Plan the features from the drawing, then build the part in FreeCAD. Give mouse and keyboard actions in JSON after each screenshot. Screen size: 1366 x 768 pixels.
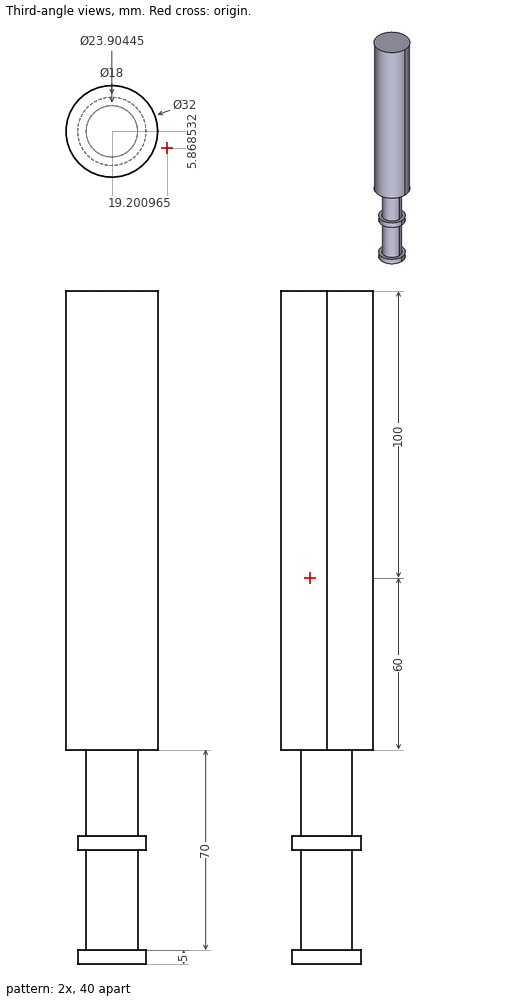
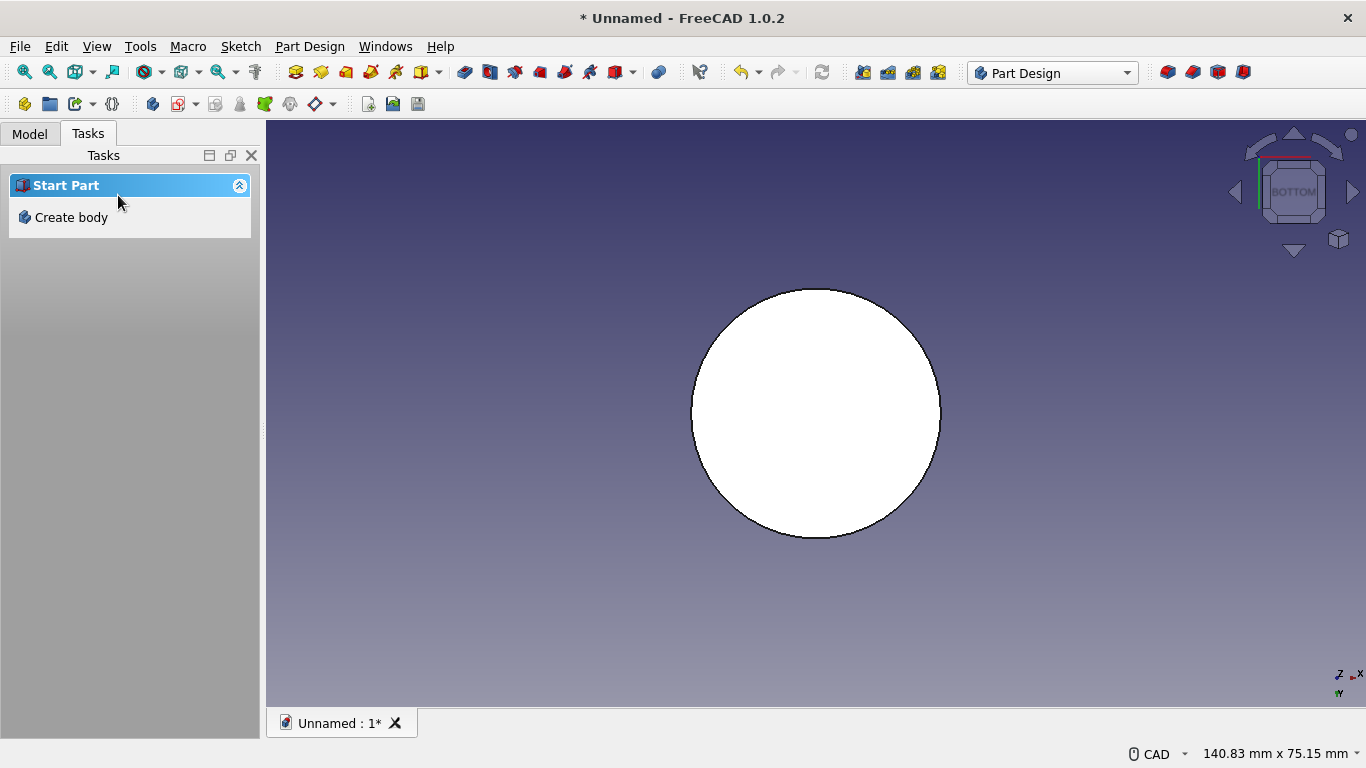
{"action": "left_click", "coordinate": [25, 72]}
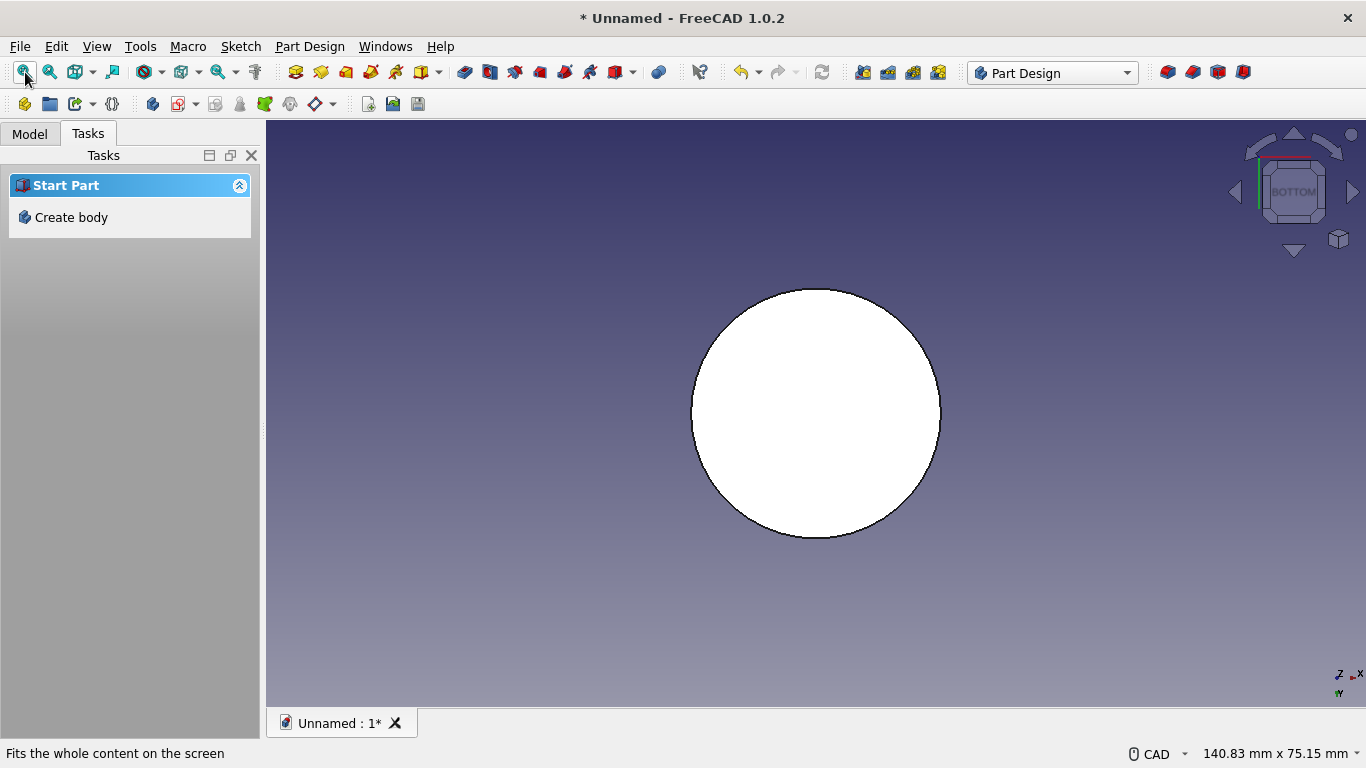
{"action": "left_click", "coordinate": [816, 412]}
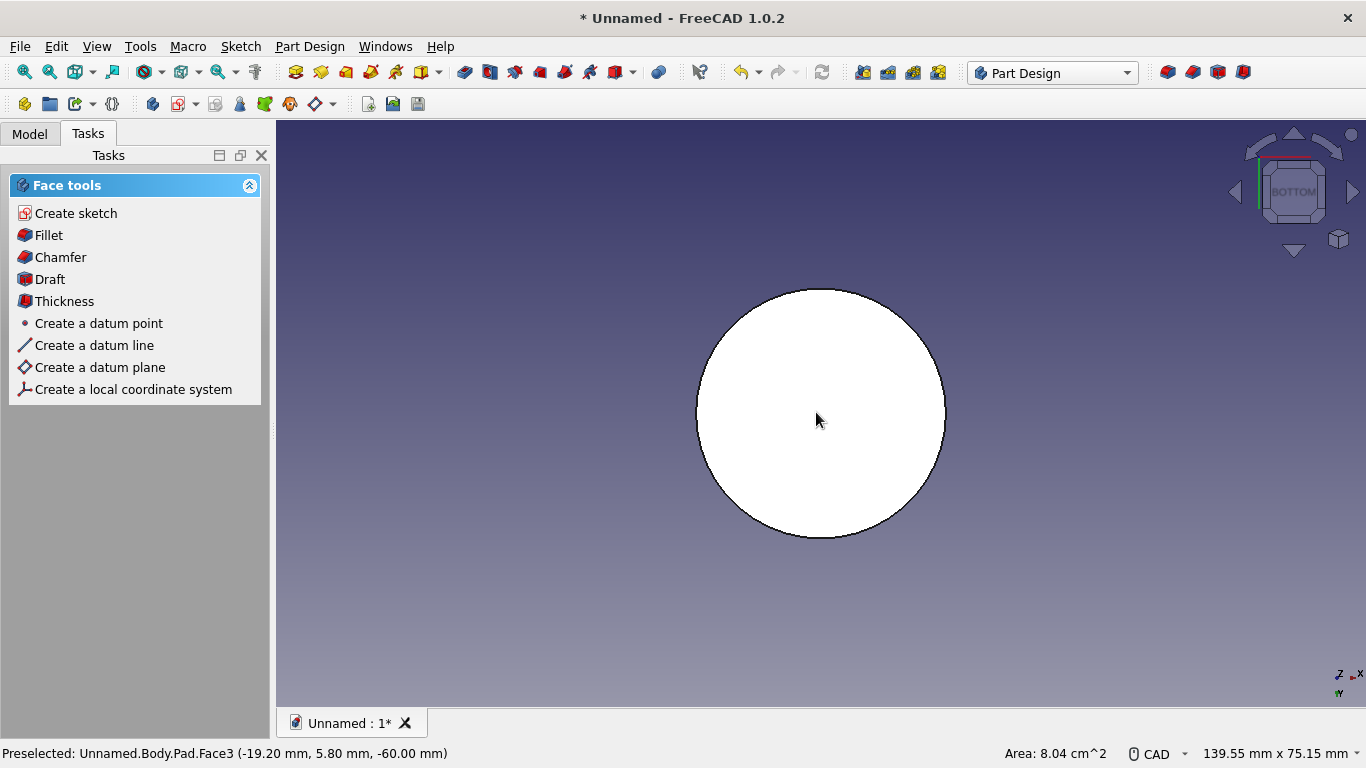
{"action": "left_click", "coordinate": [178, 104]}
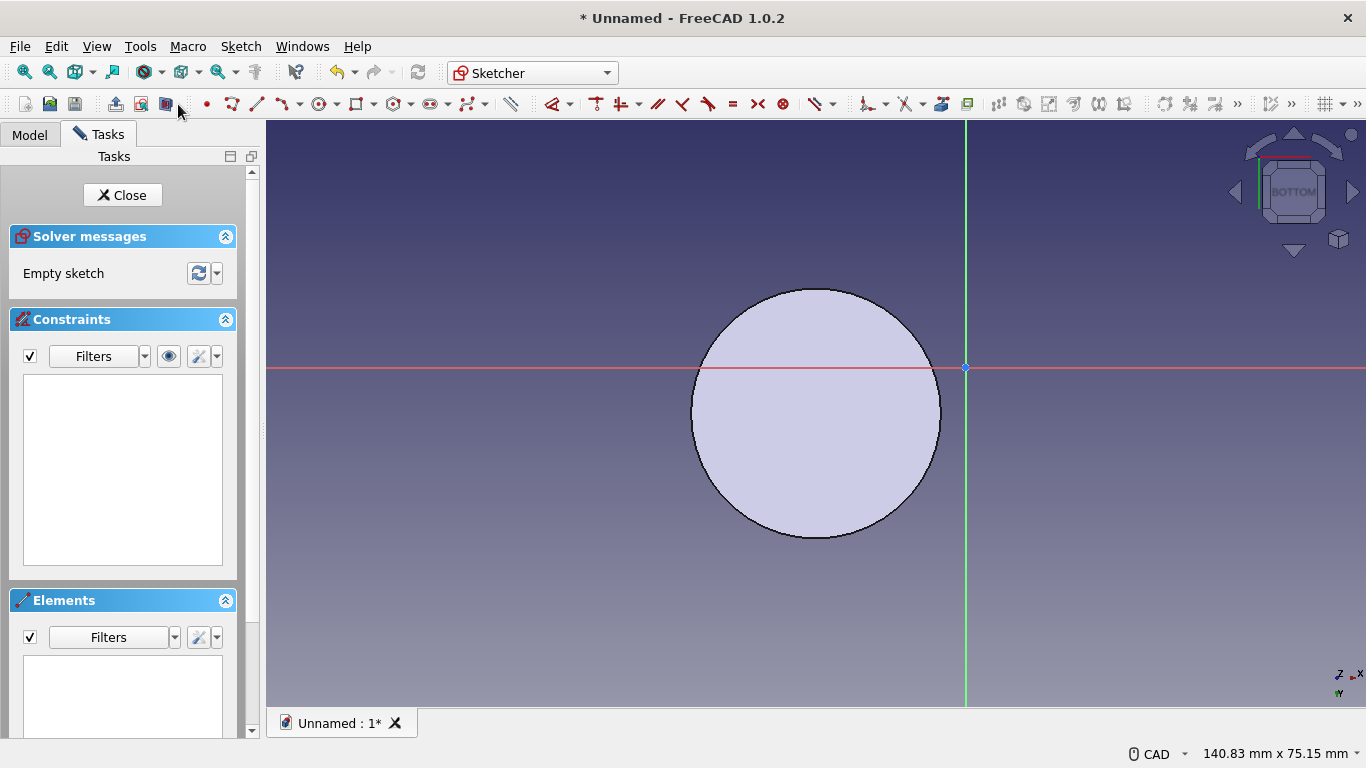
{"action": "scroll", "coordinate": [919, 413], "scroll_direction": "up", "scroll_amount": 5}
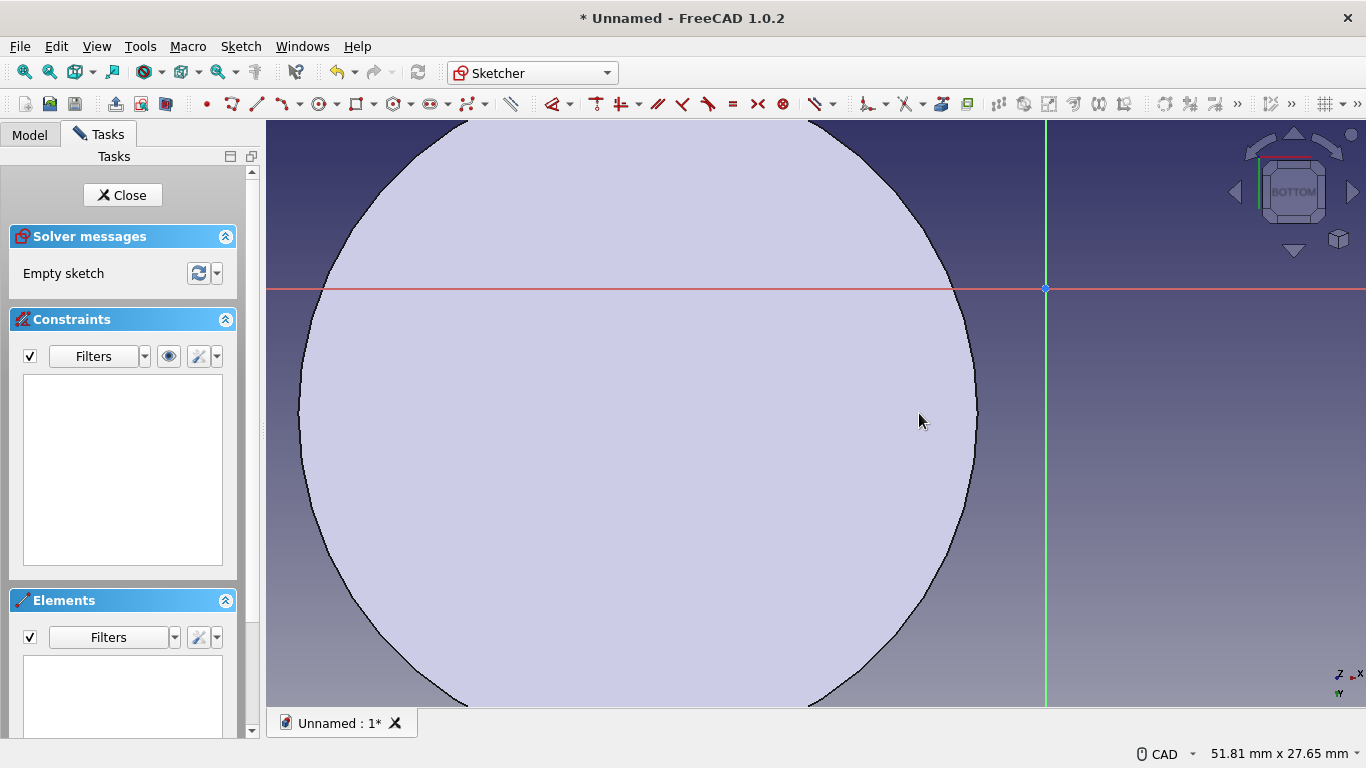
{"action": "key", "text": "g c"}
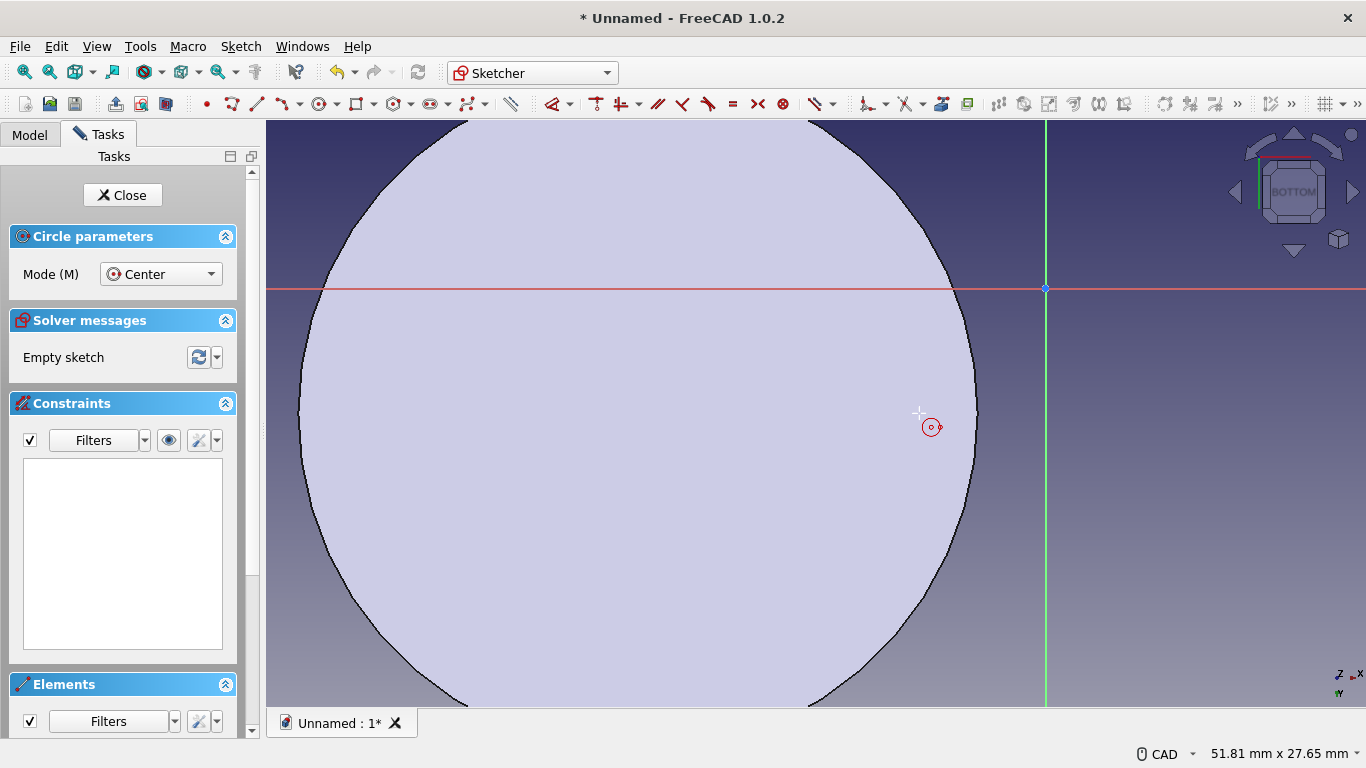
{"action": "left_click", "coordinate": [638, 413]}
{"action": "mouse_move", "coordinate": [773, 549]}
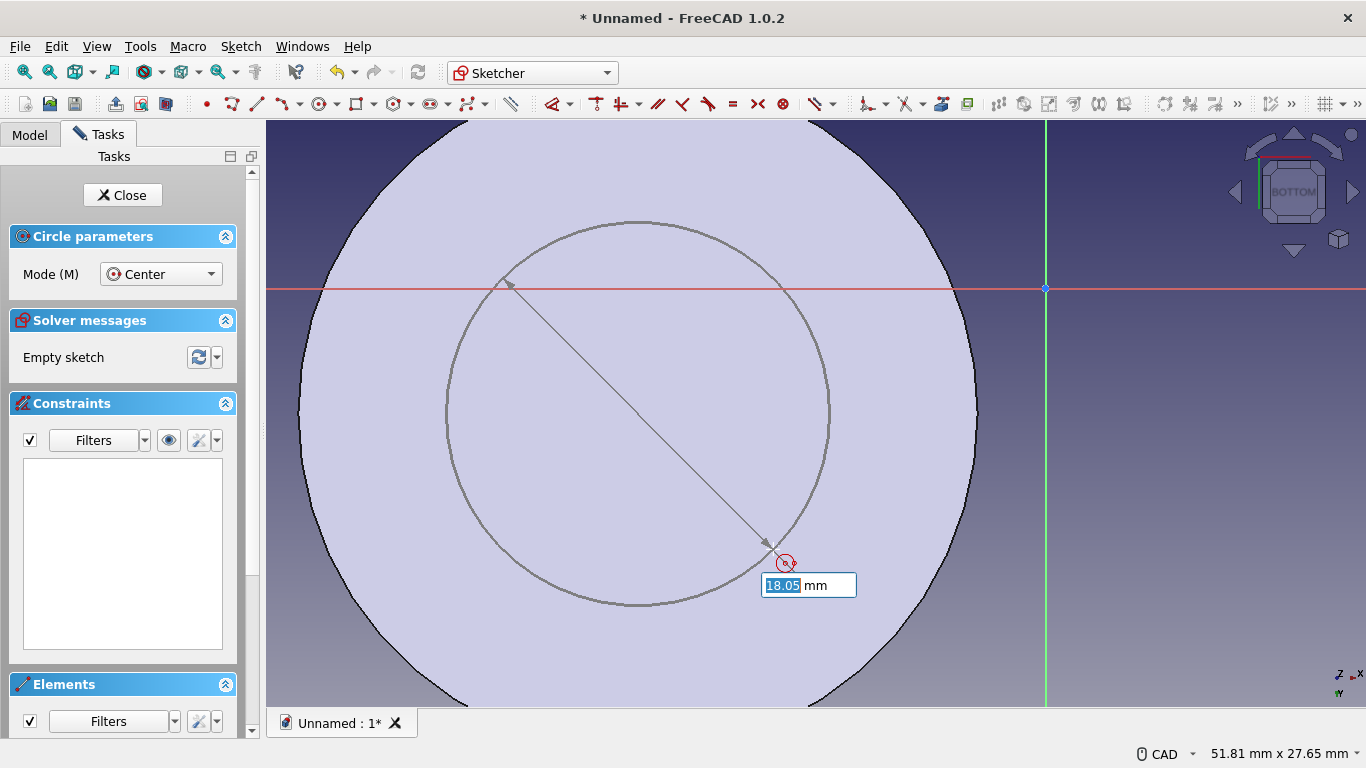
{"action": "type", "text": "18"}
{"action": "key", "text": "Return"}
{"action": "key", "text": "Escape"}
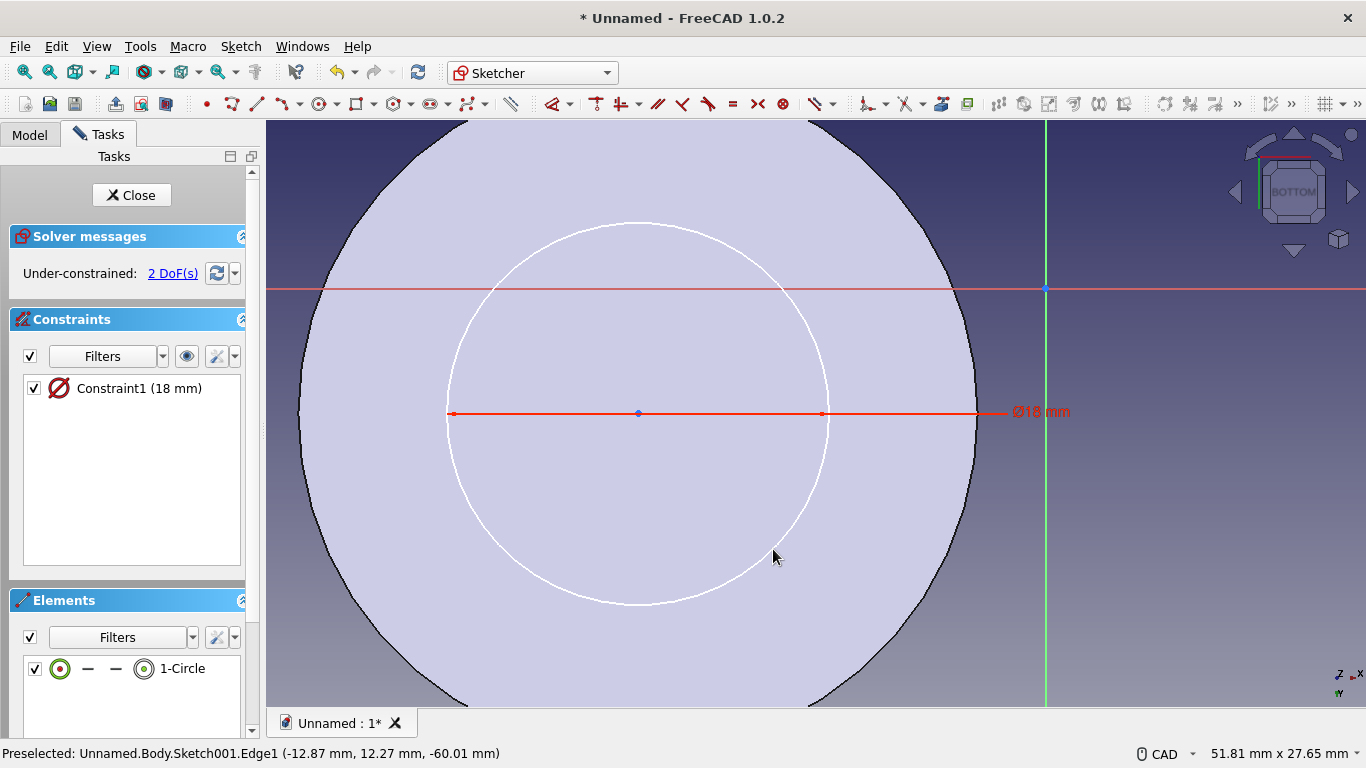
{"action": "key", "text": "d"}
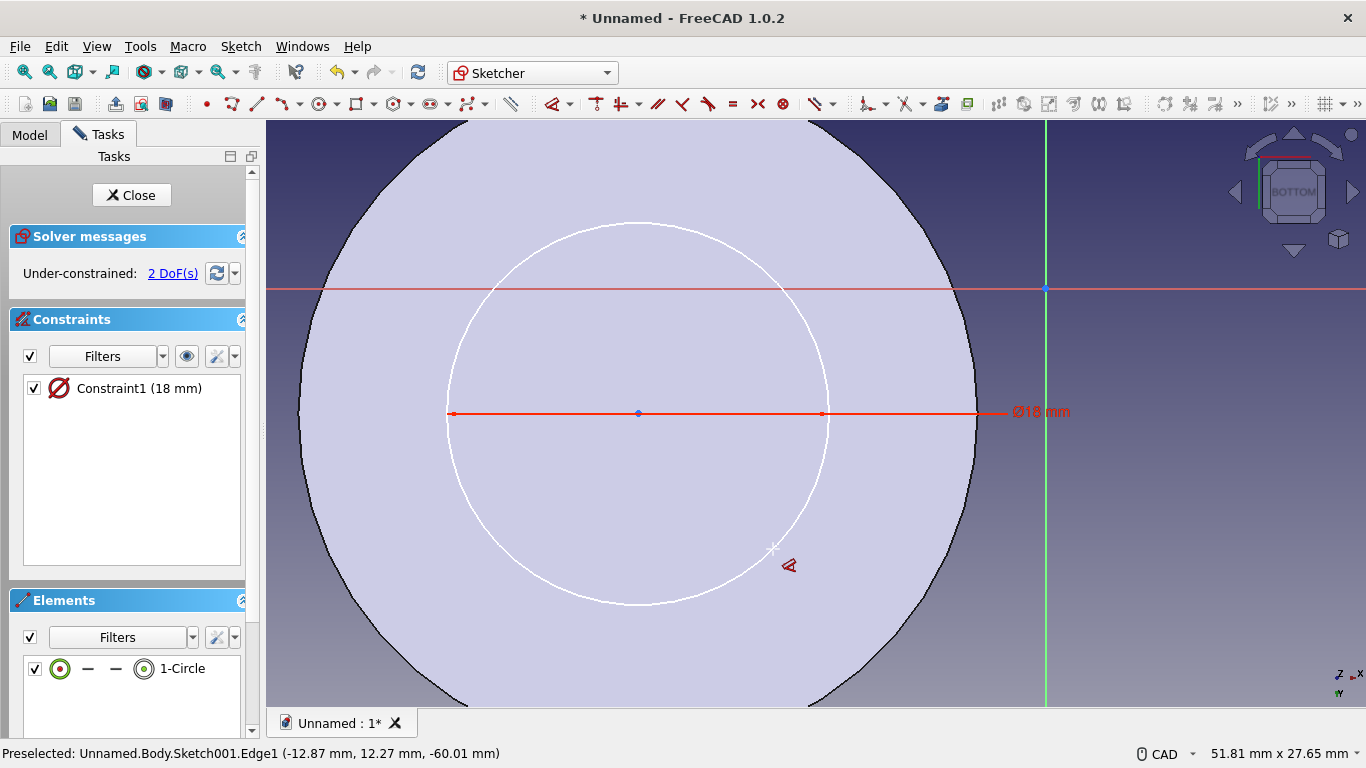
{"action": "left_click", "coordinate": [638, 414]}
{"action": "left_click", "coordinate": [1080, 351]}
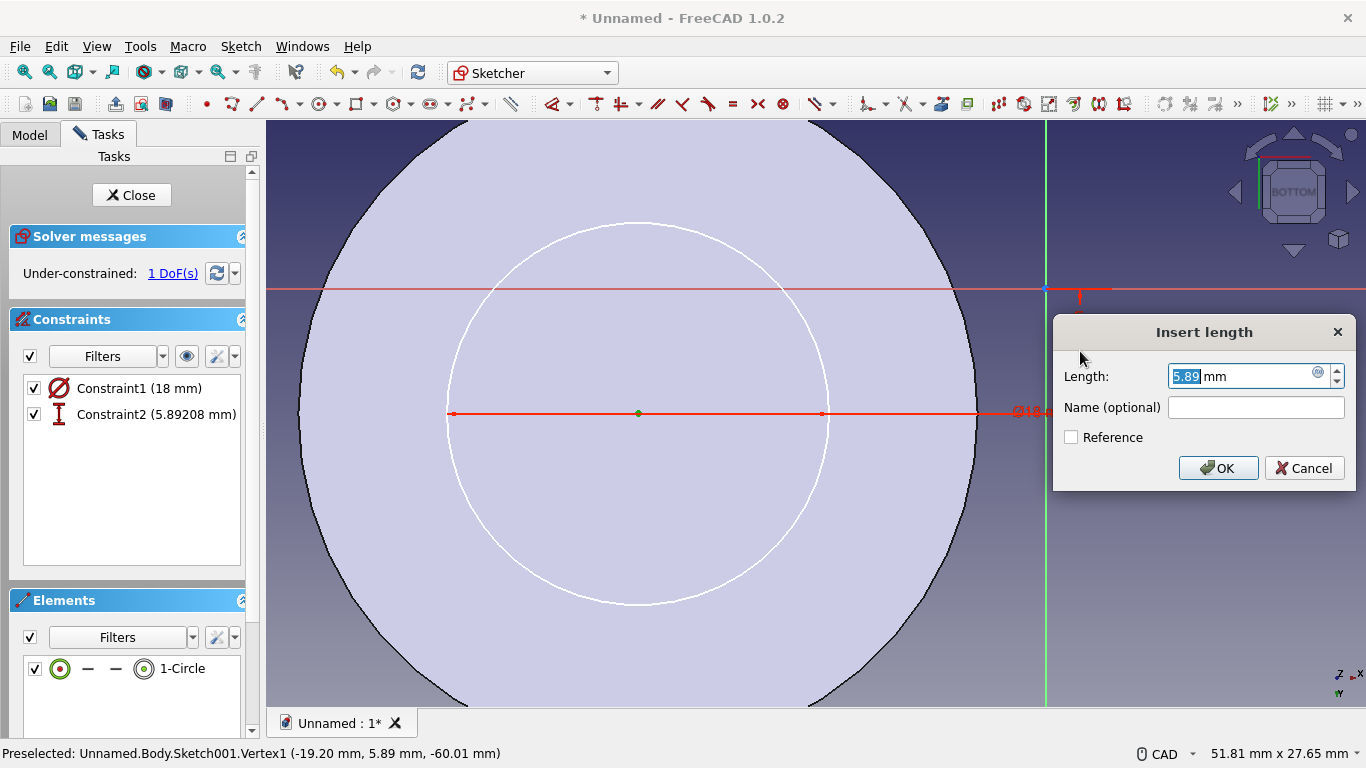
{"action": "type", "text": "5.868532"}
{"action": "key", "text": "Return"}